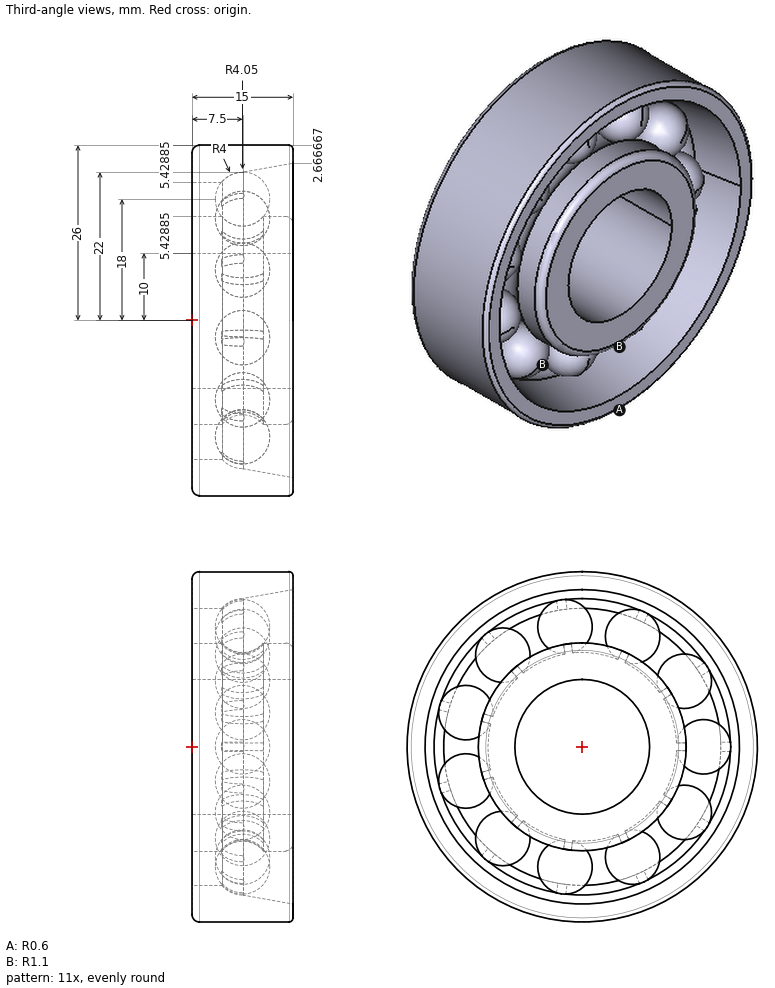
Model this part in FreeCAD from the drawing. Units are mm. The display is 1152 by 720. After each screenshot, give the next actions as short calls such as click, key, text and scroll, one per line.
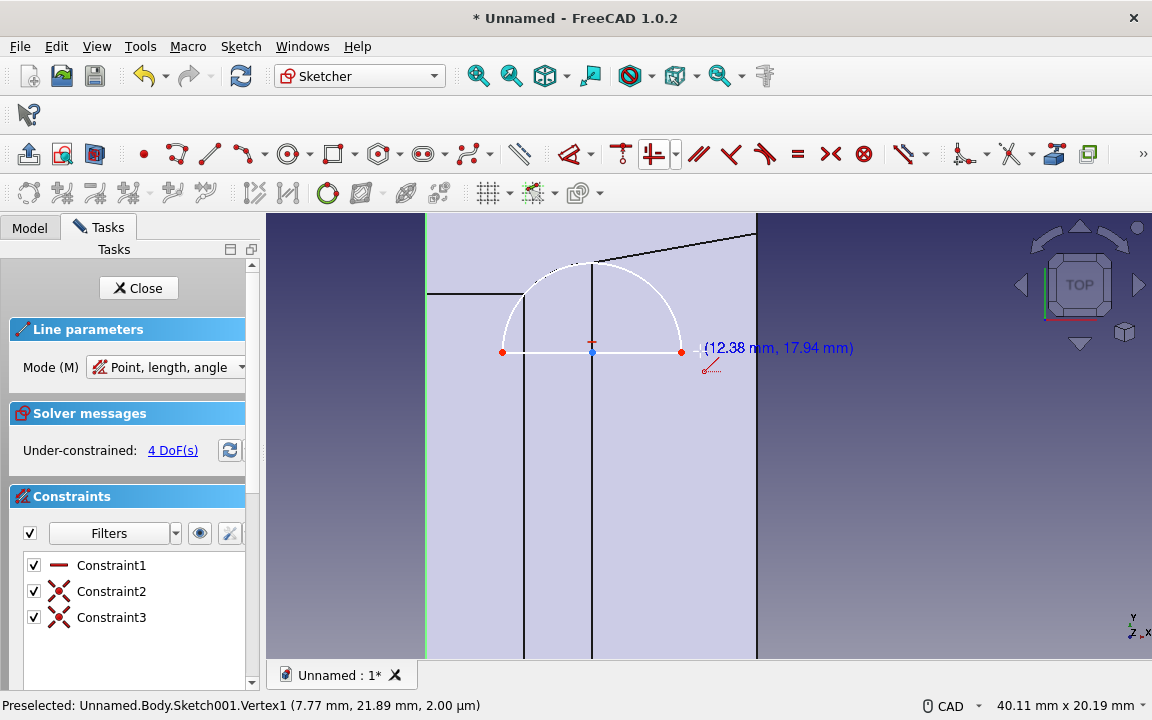
click(699, 351)
click(753, 351)
key(Escape)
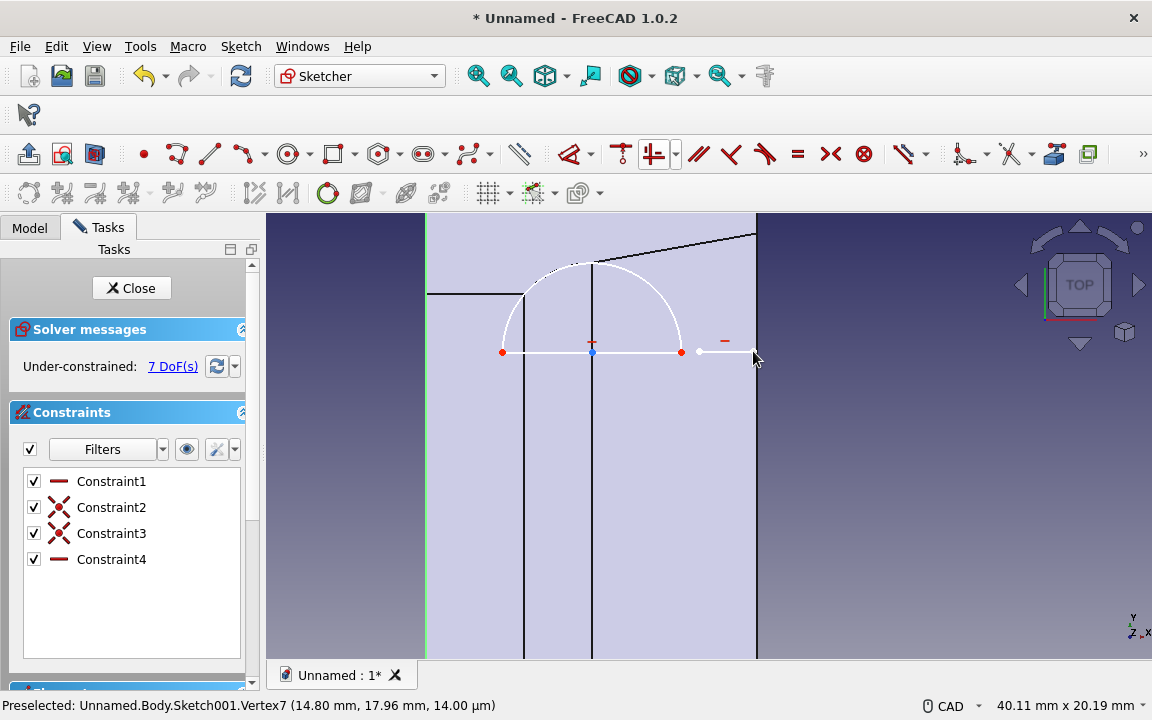
click(715, 352)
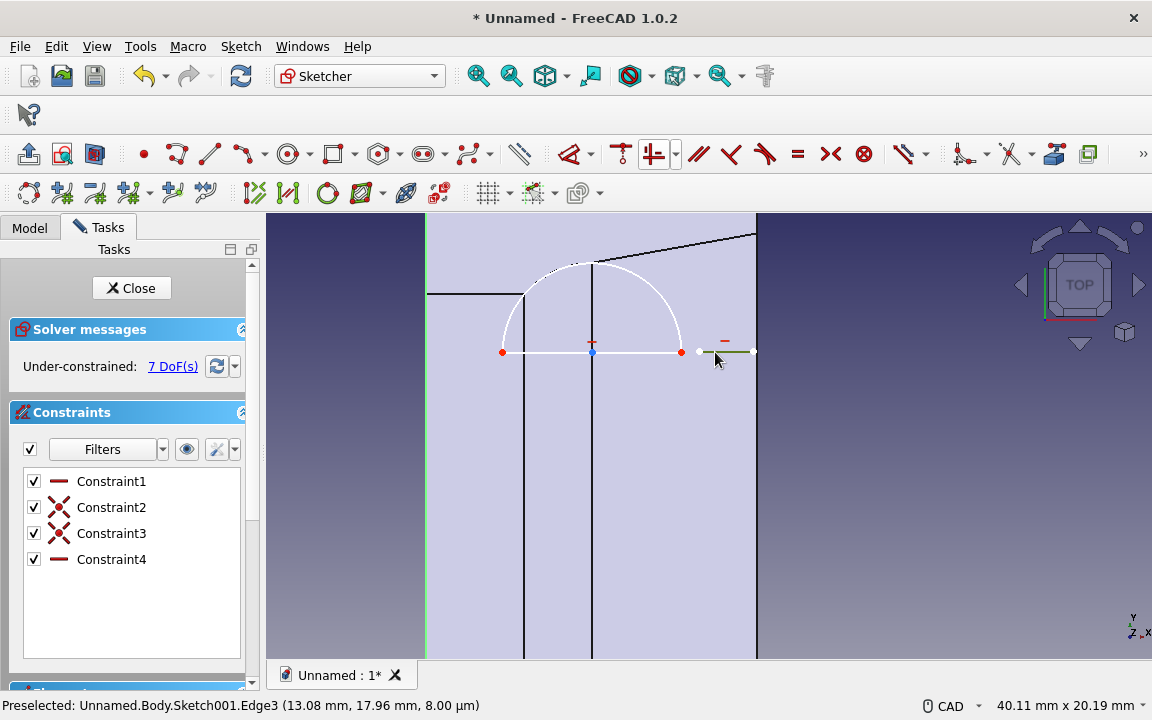
click(520, 154)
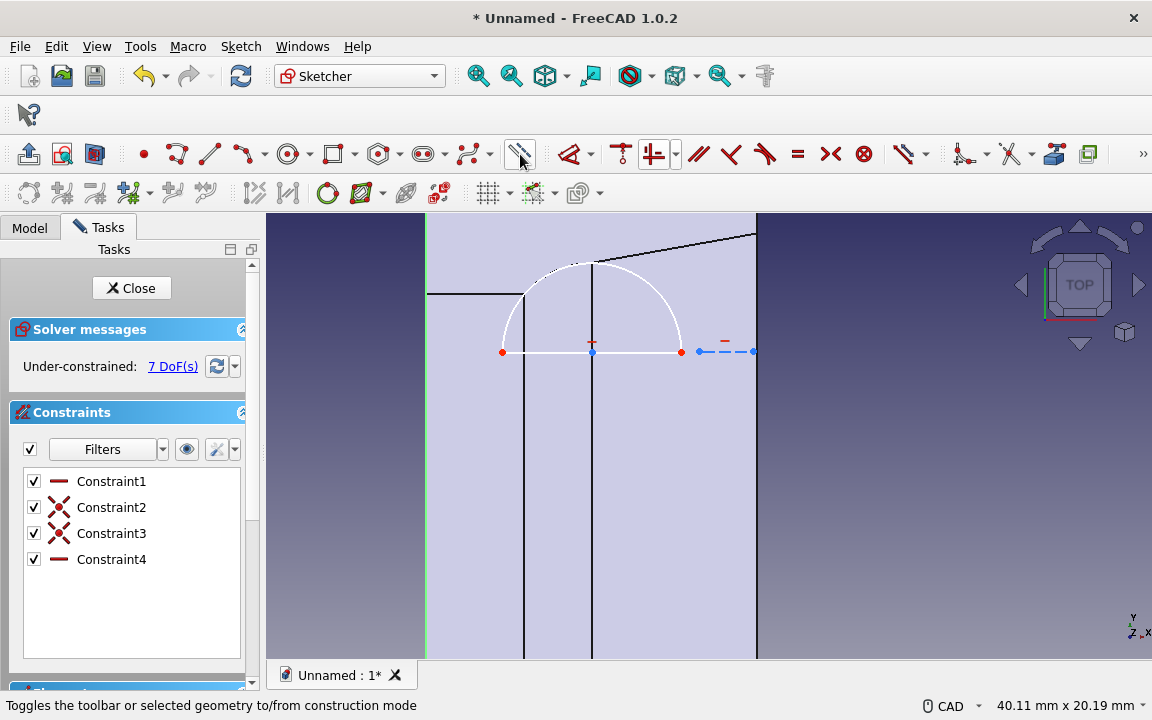
click(568, 154)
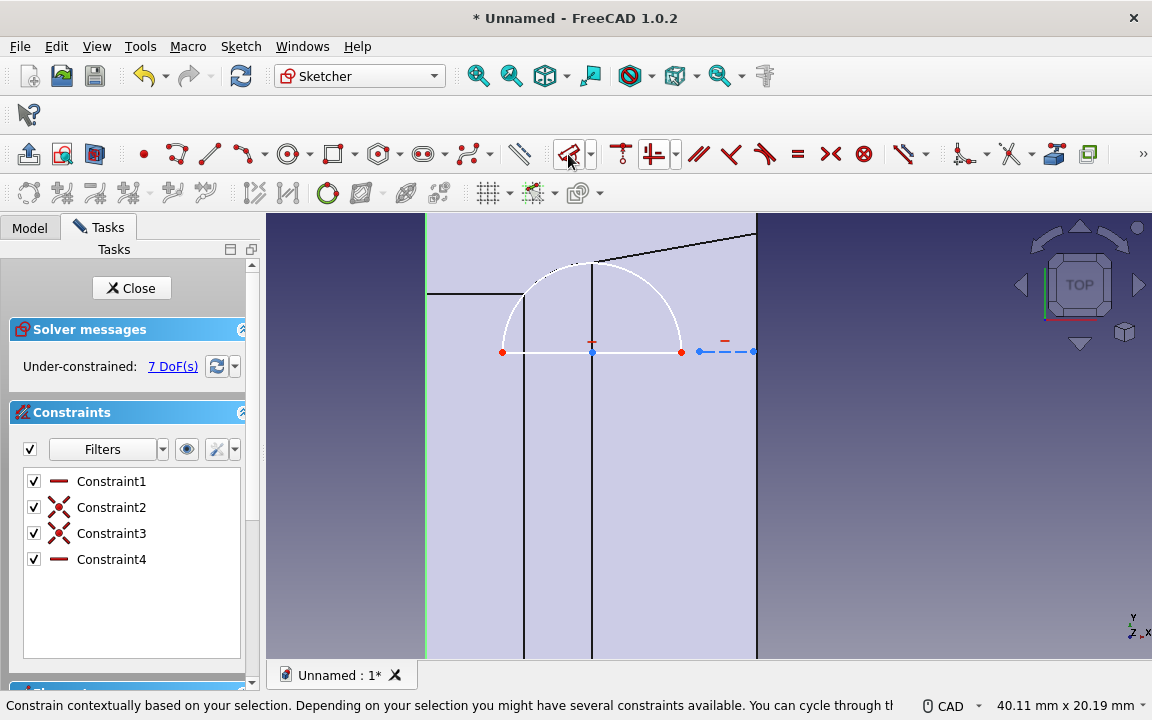
click(645, 280)
click(664, 254)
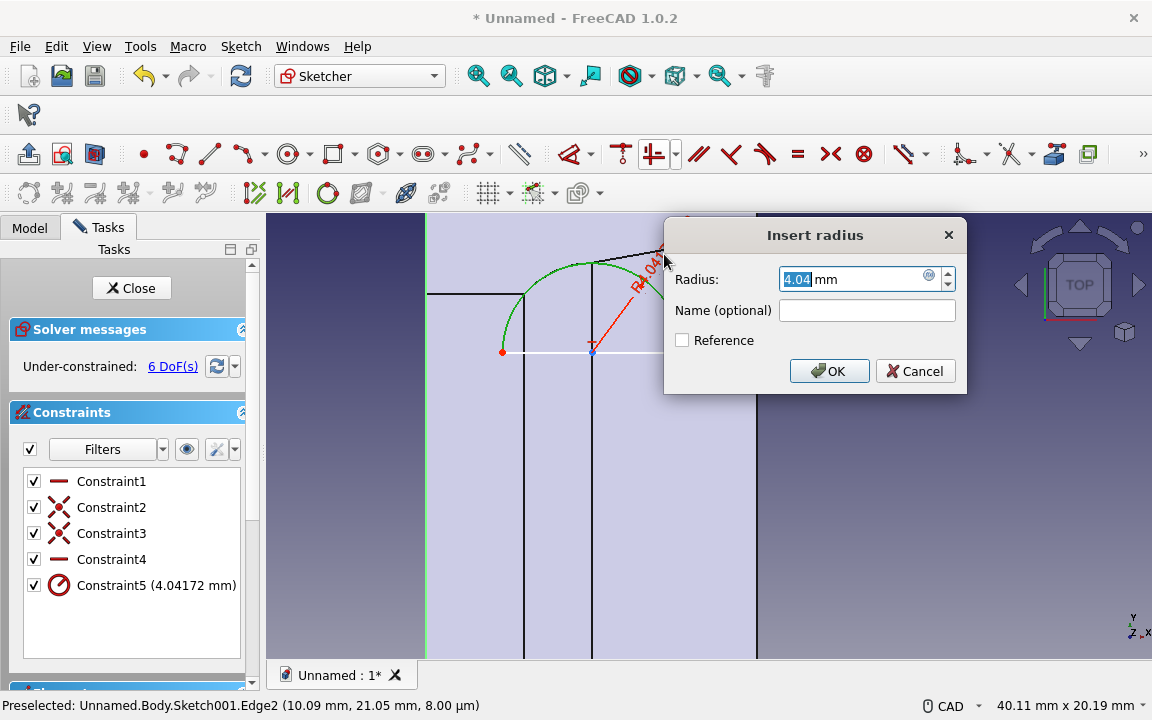
text(4.05)
key(Return)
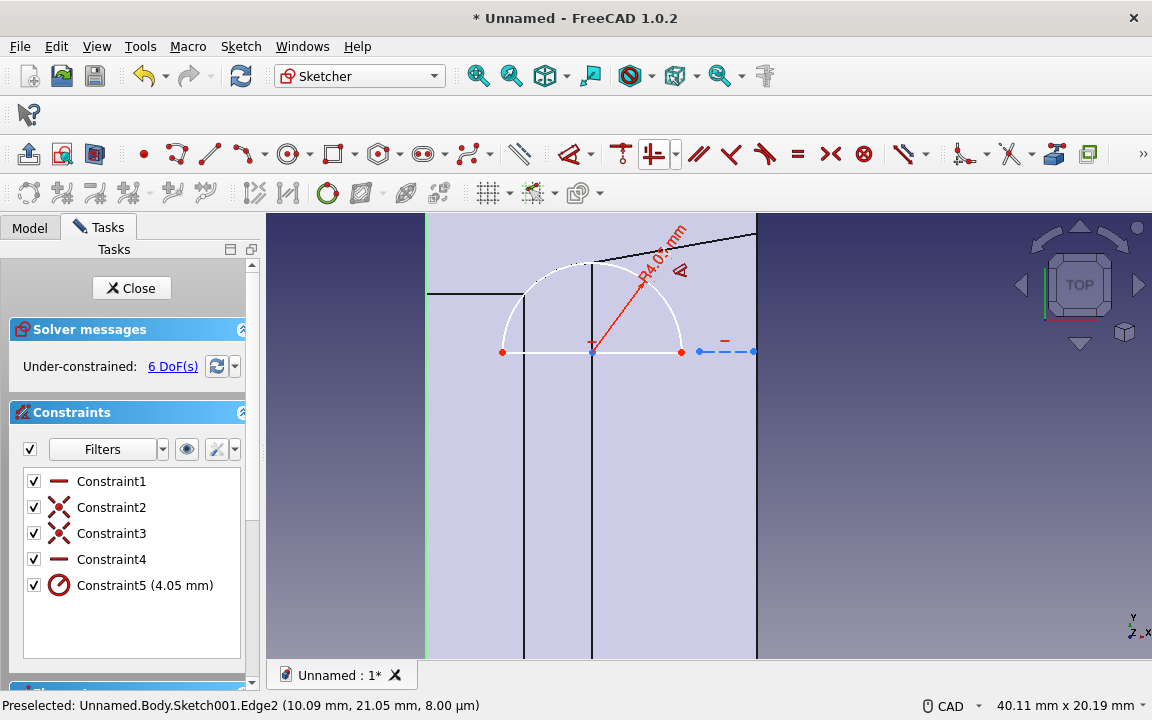
click(503, 353)
click(392, 492)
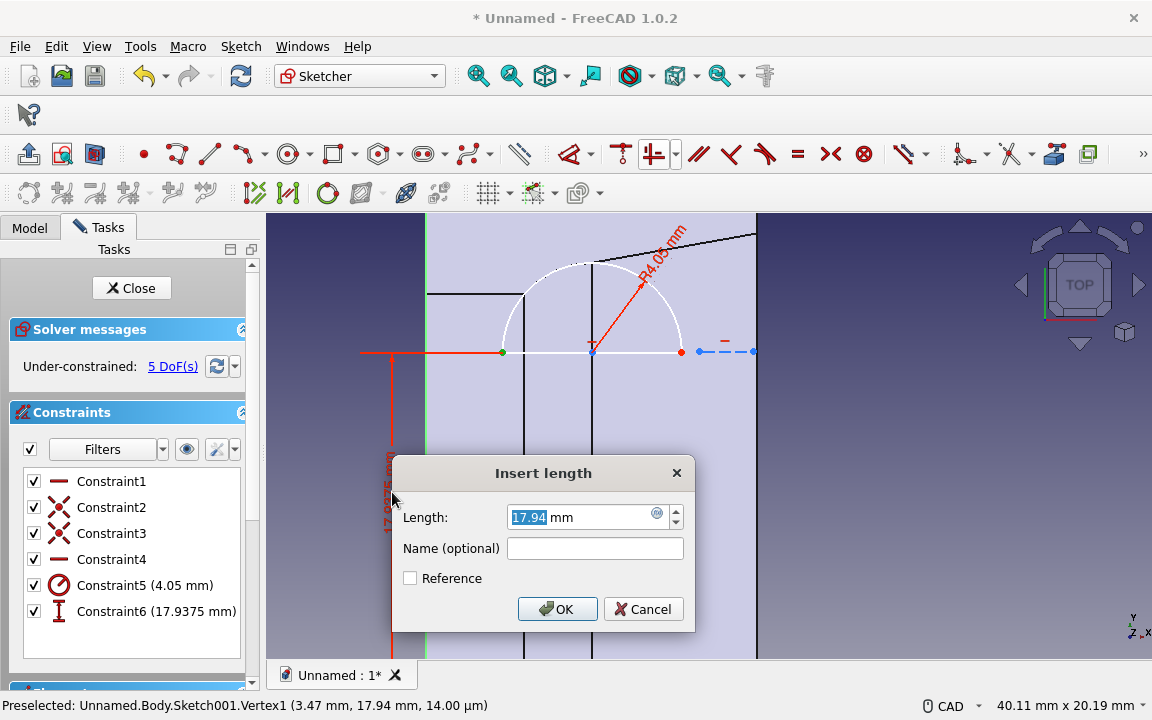
text(18)
key(Return)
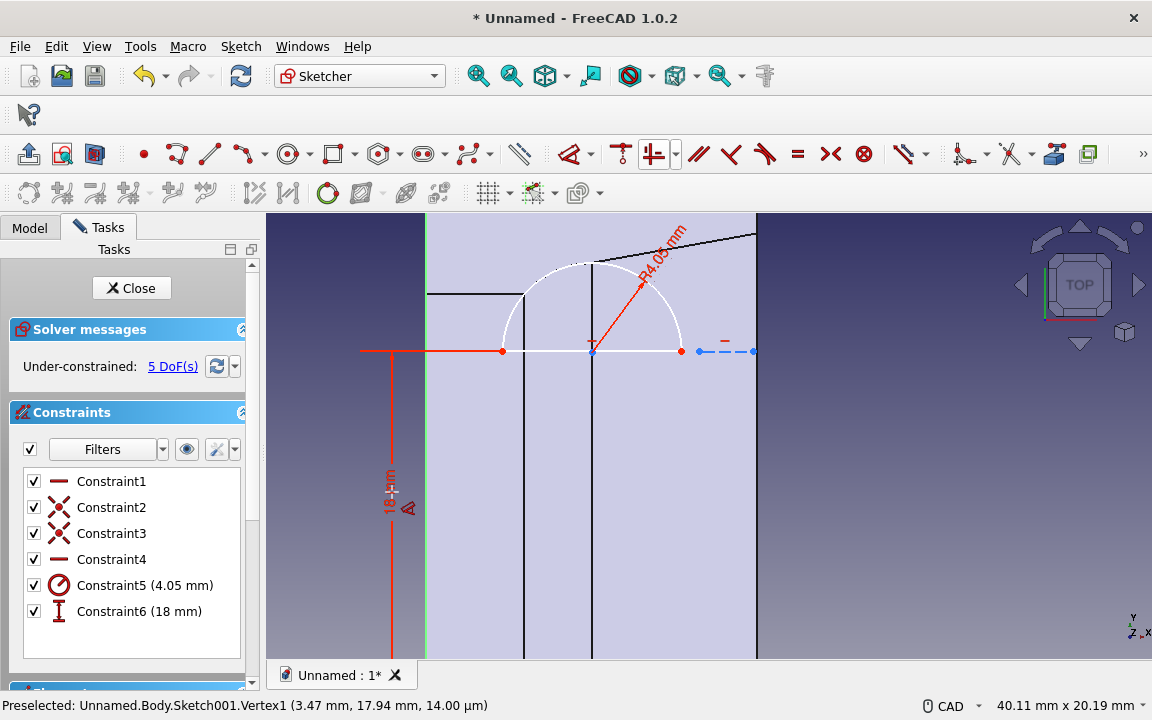
click(699, 352)
click(392, 427)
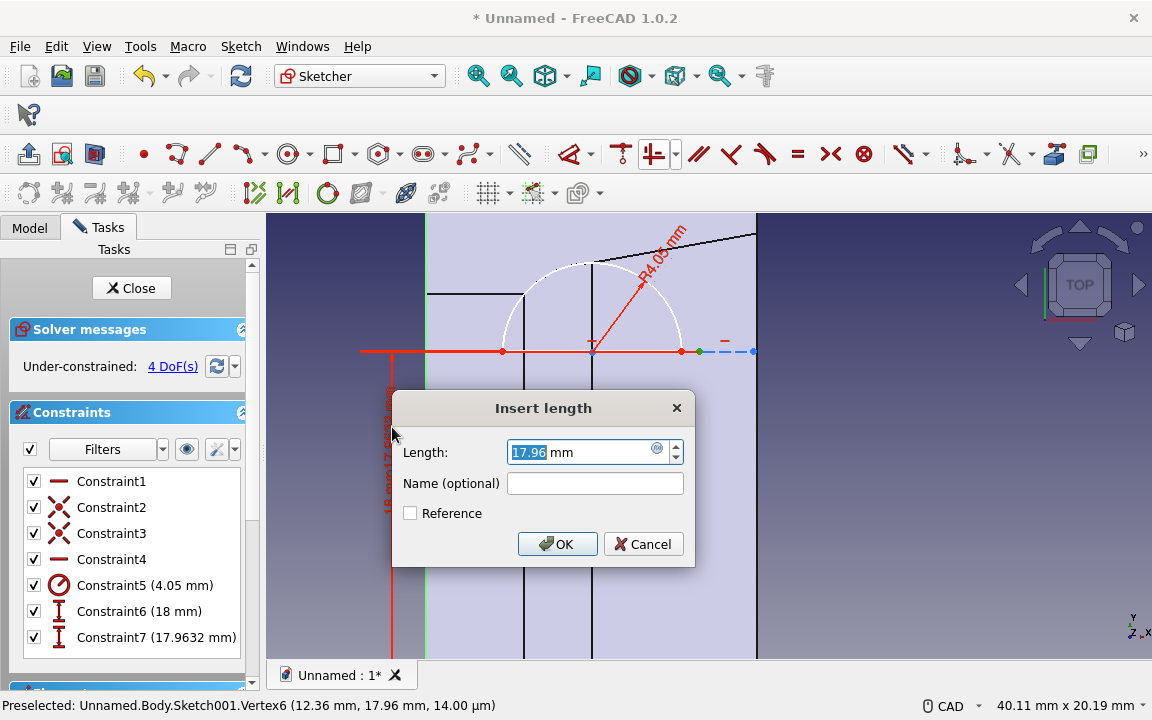
text(18)
key(Return)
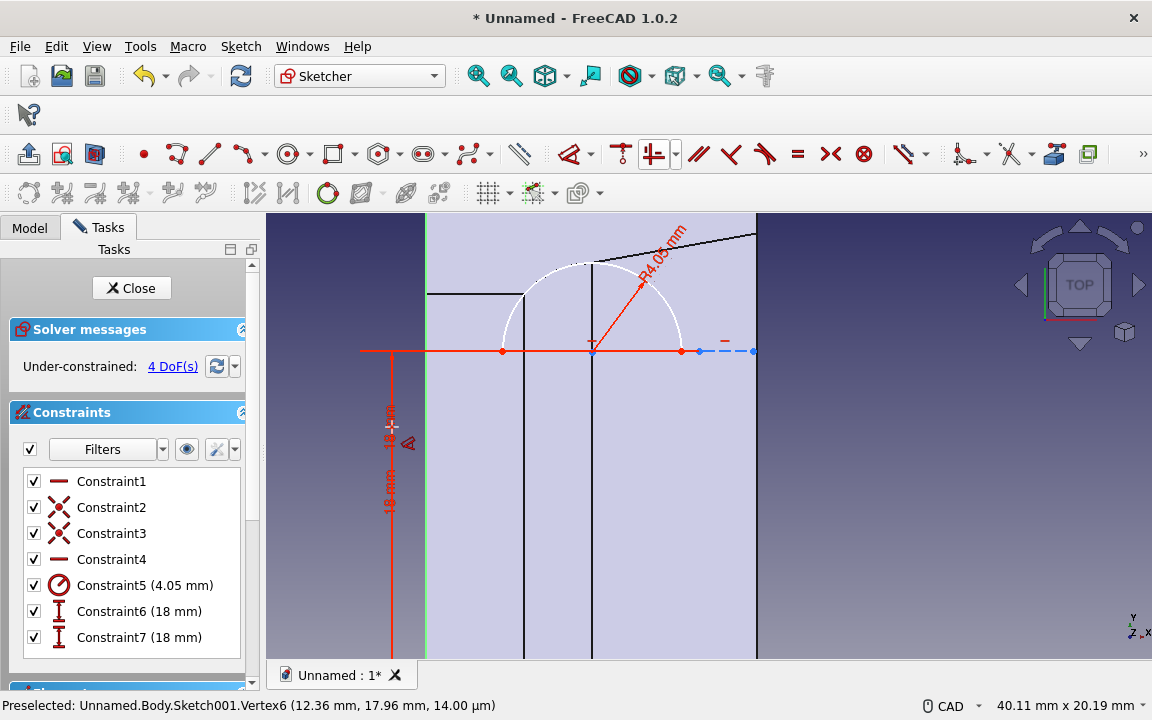
click(592, 353)
click(392, 556)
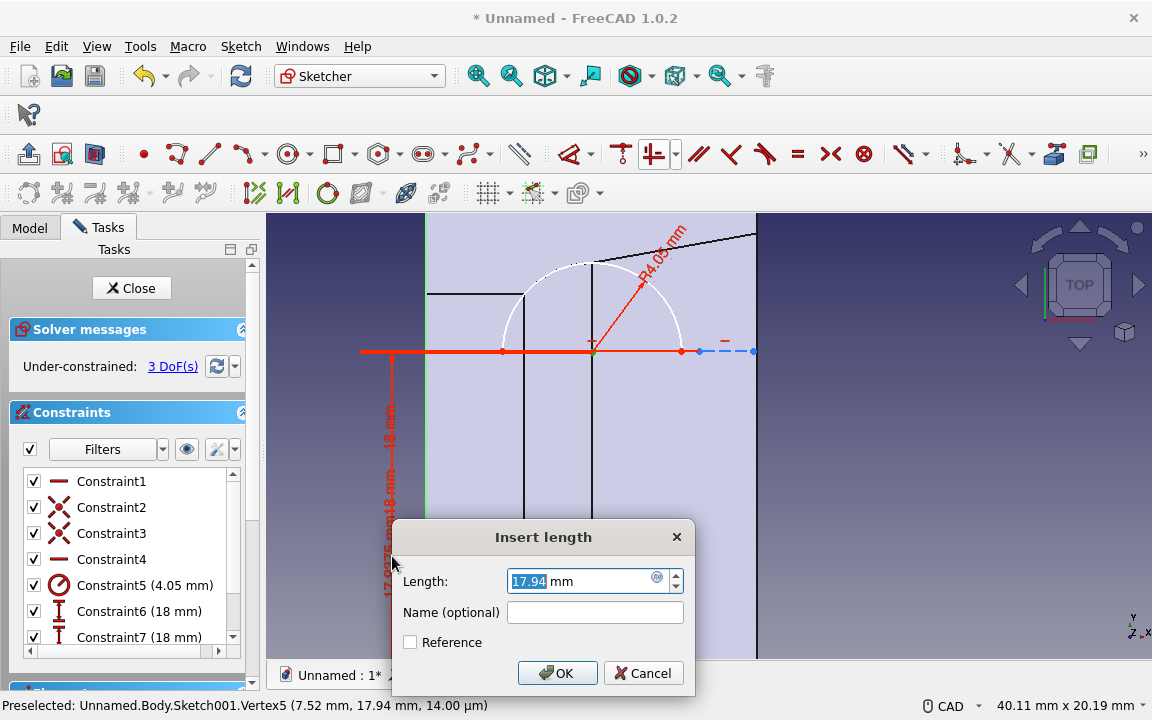
text(18)
key(Return)